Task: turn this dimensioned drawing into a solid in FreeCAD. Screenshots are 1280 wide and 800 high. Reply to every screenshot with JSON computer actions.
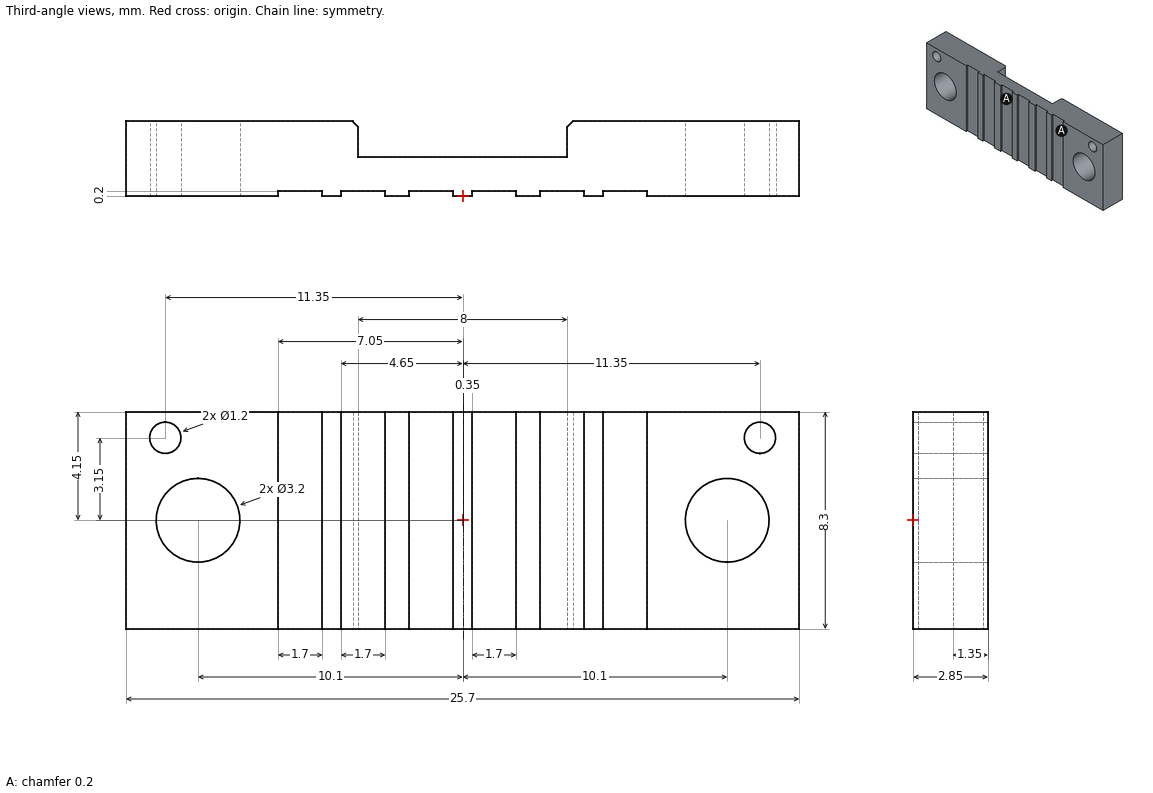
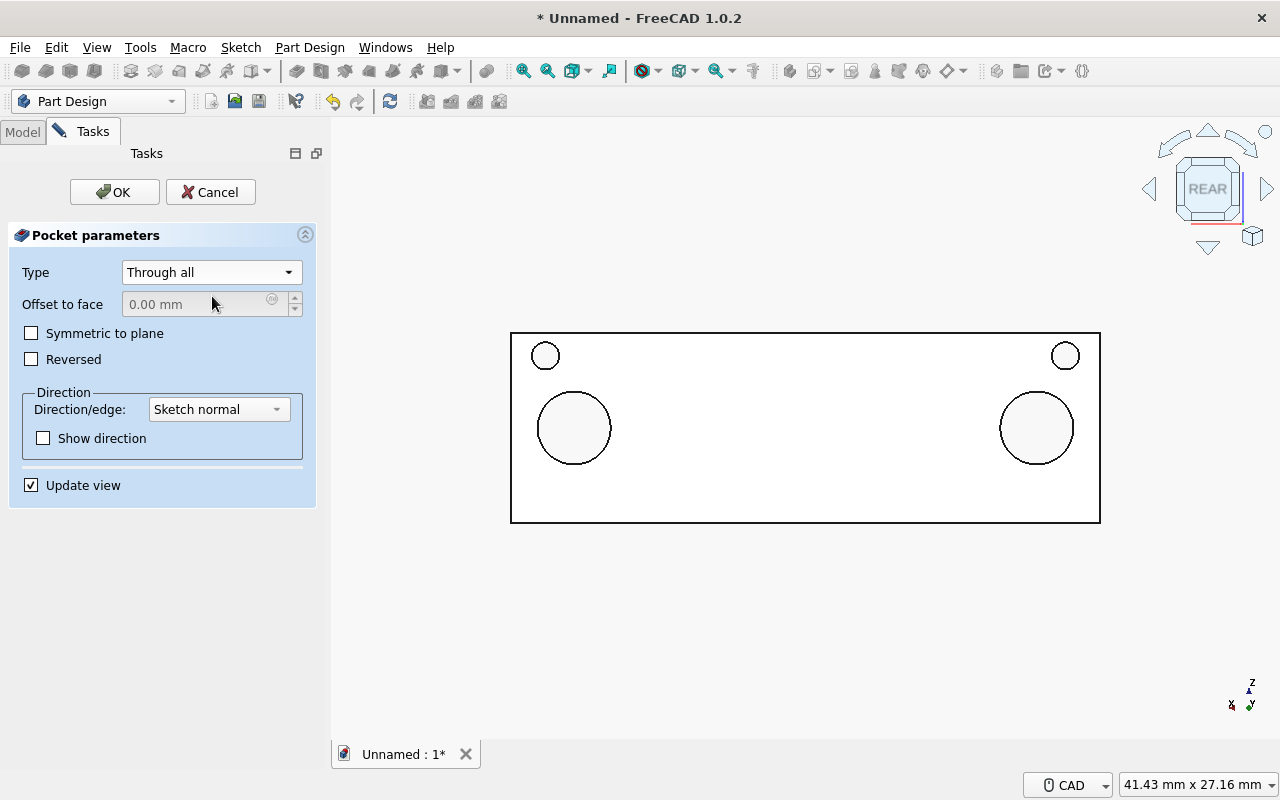
{"action": "left_click", "coordinate": [115, 192]}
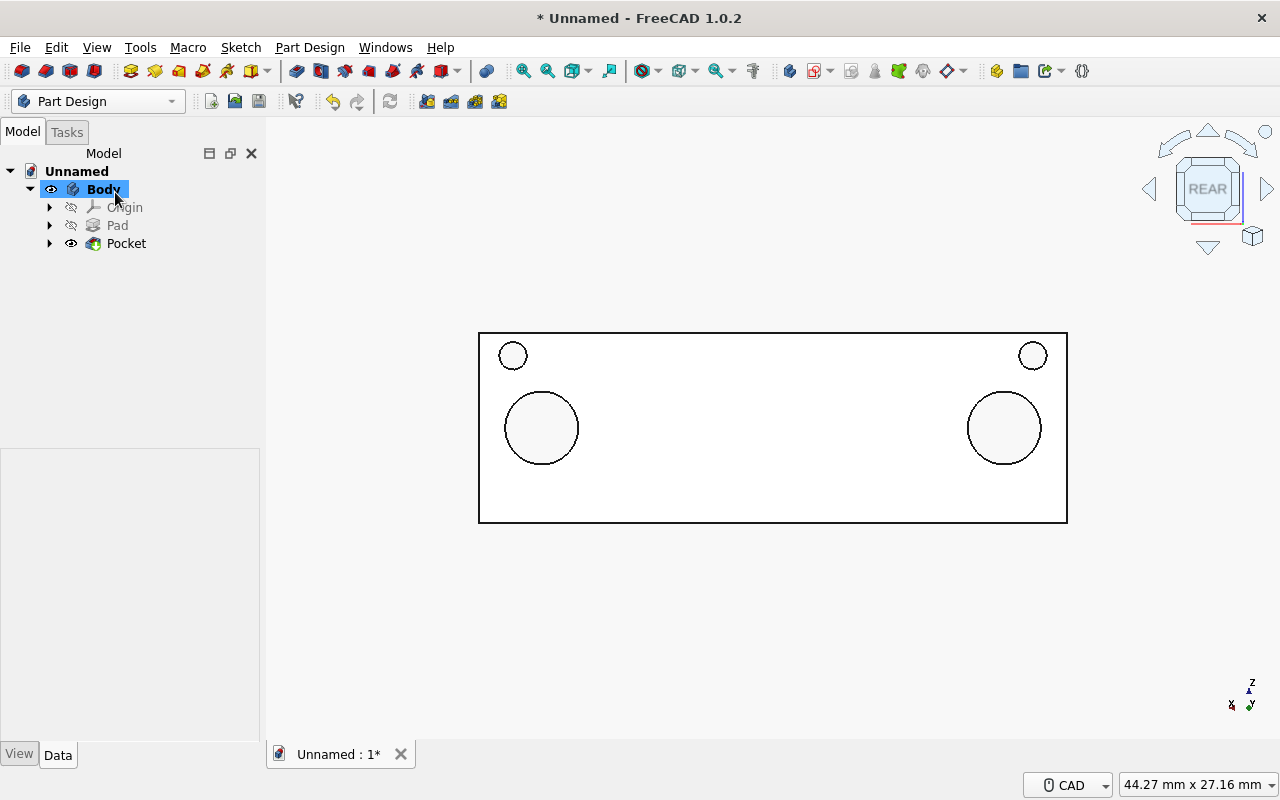
{"action": "key", "text": "0"}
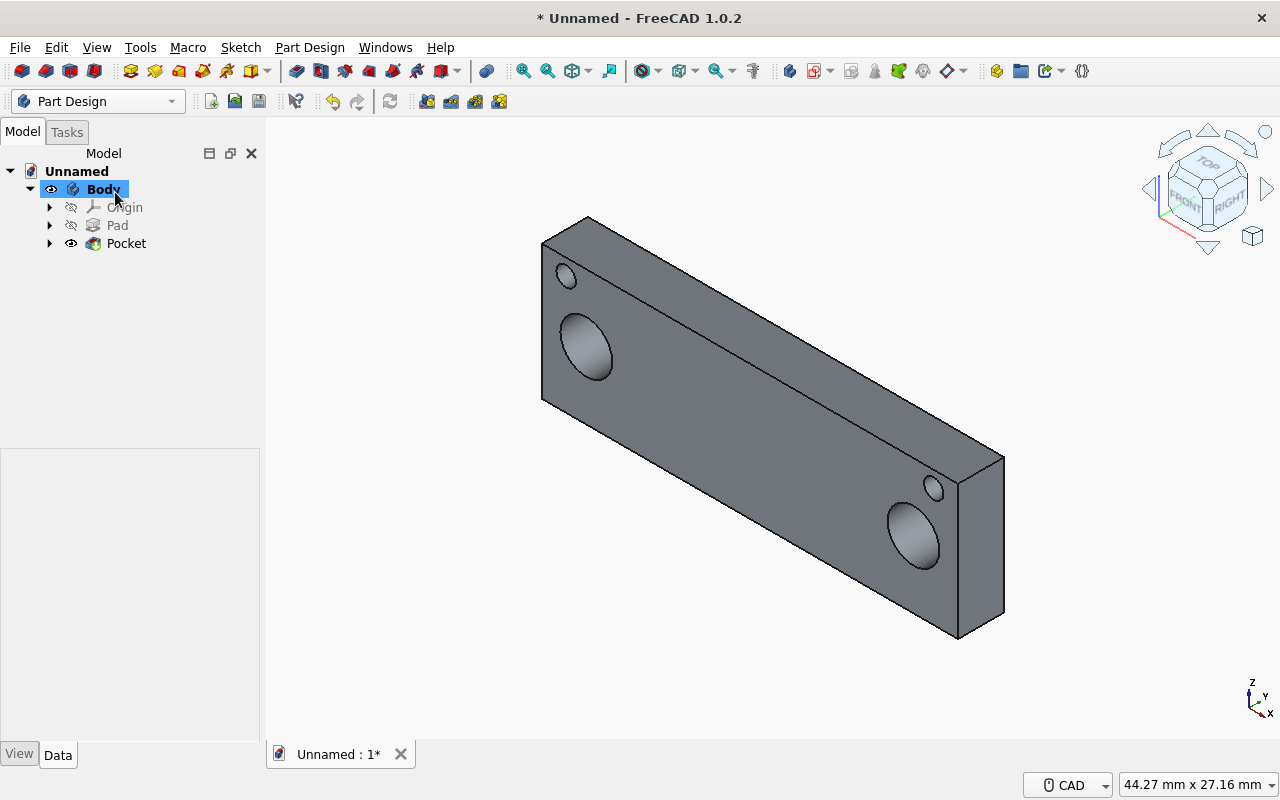
{"action": "left_click", "coordinate": [809, 475]}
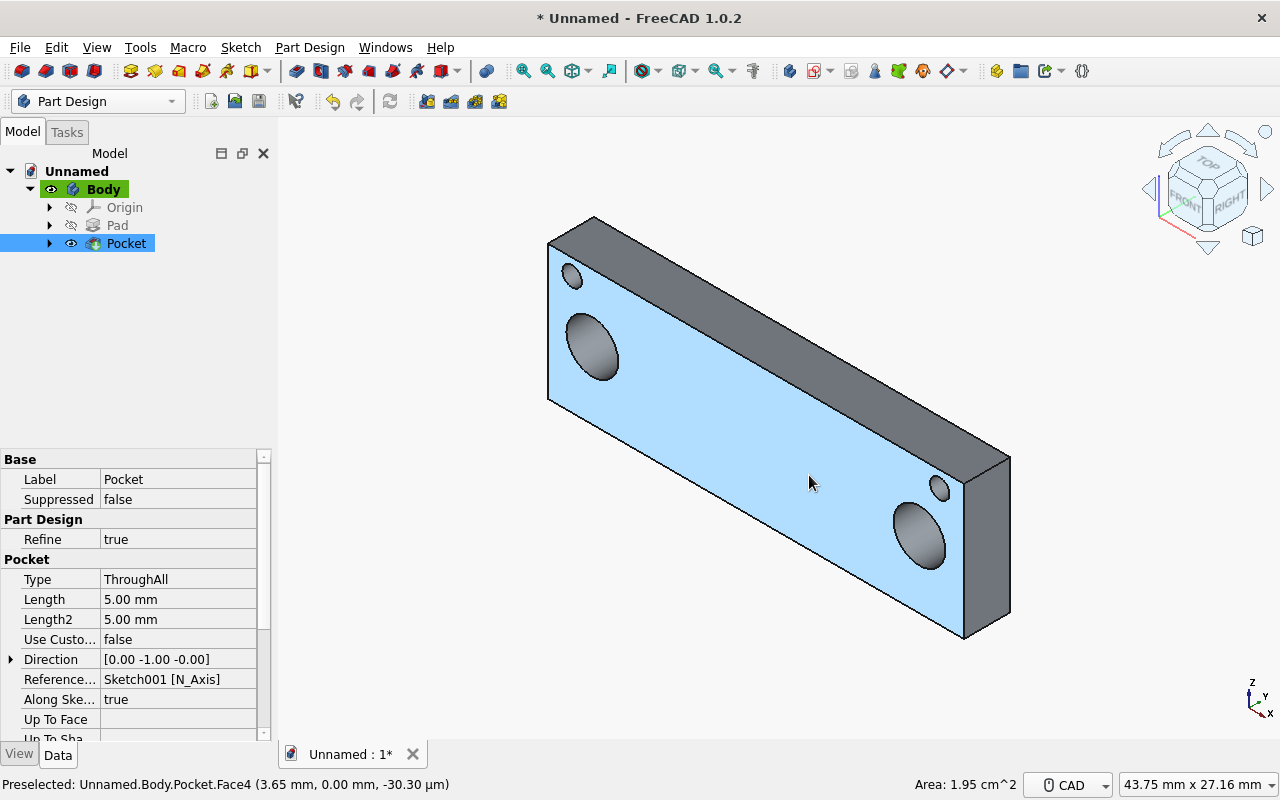
{"action": "left_click", "coordinate": [814, 72]}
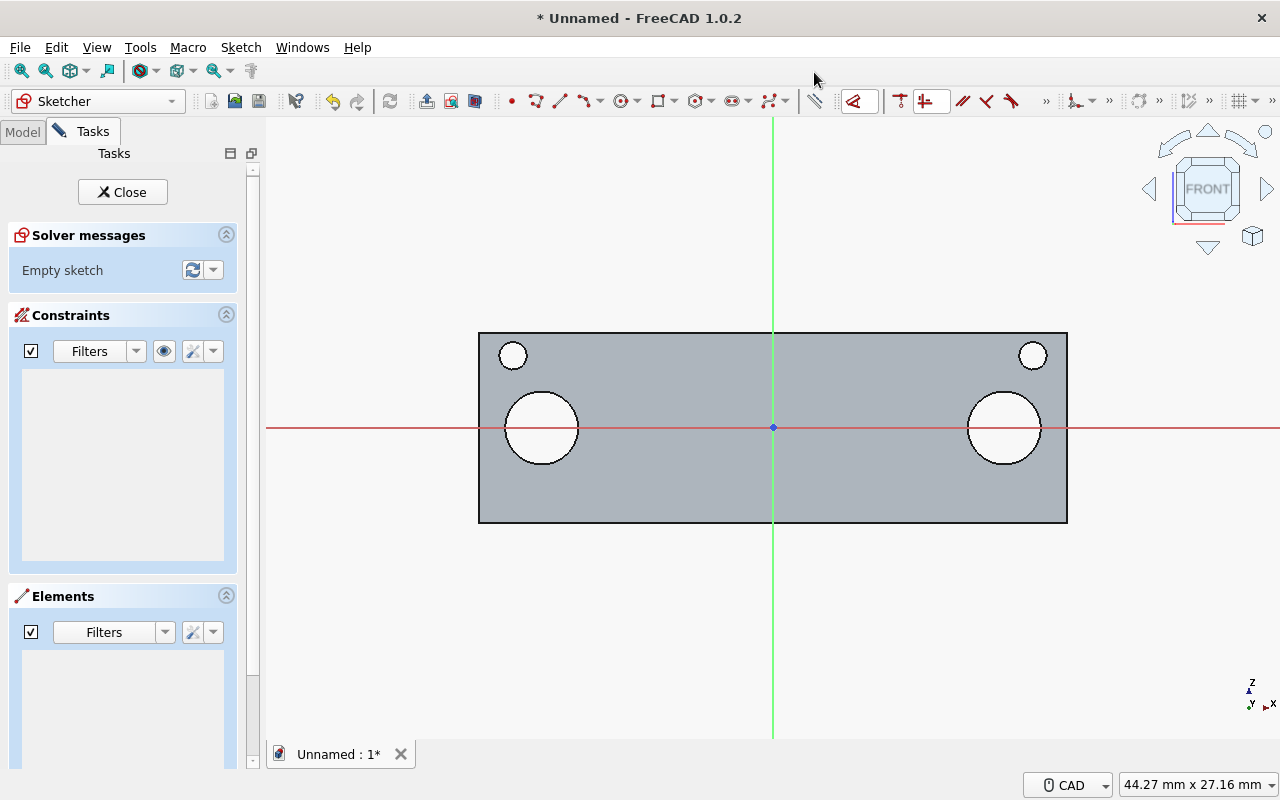
{"action": "scroll", "coordinate": [856, 428], "scroll_direction": "up", "scroll_amount": 3}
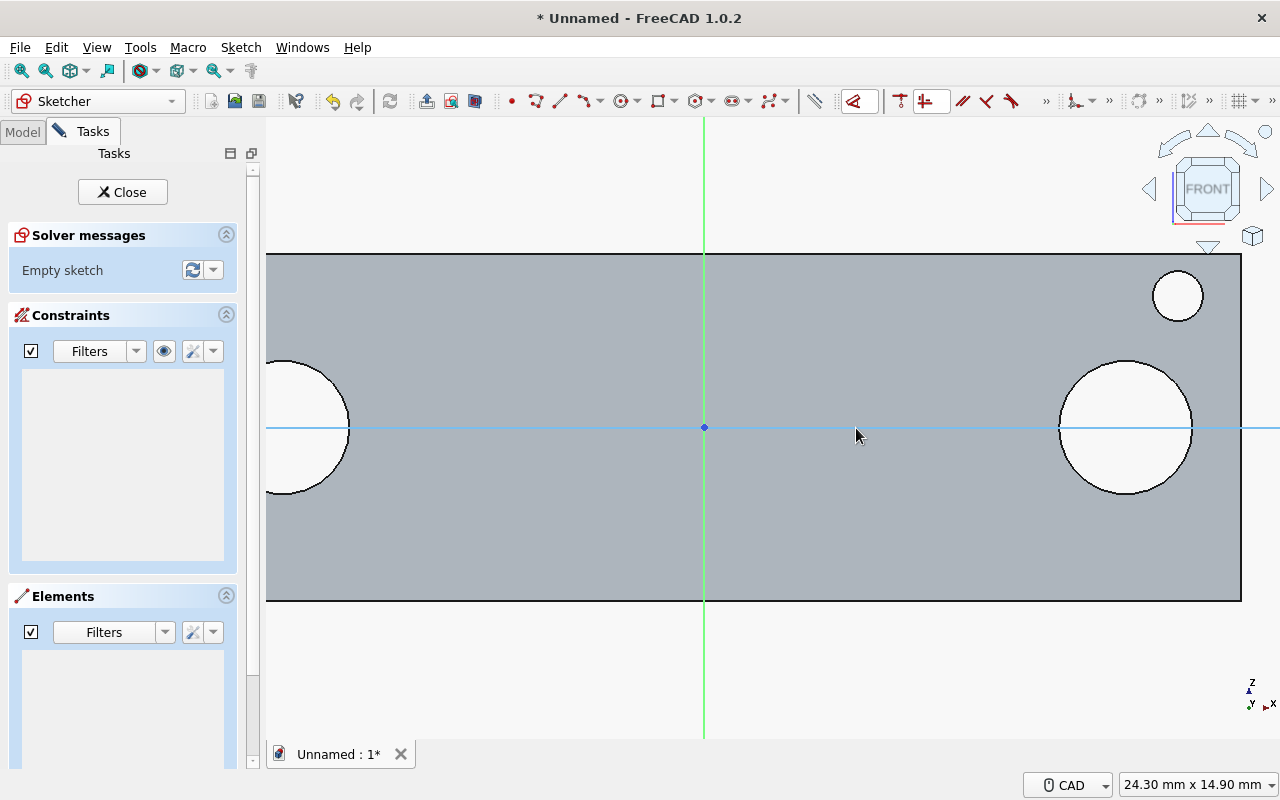
{"action": "key", "text": "g r"}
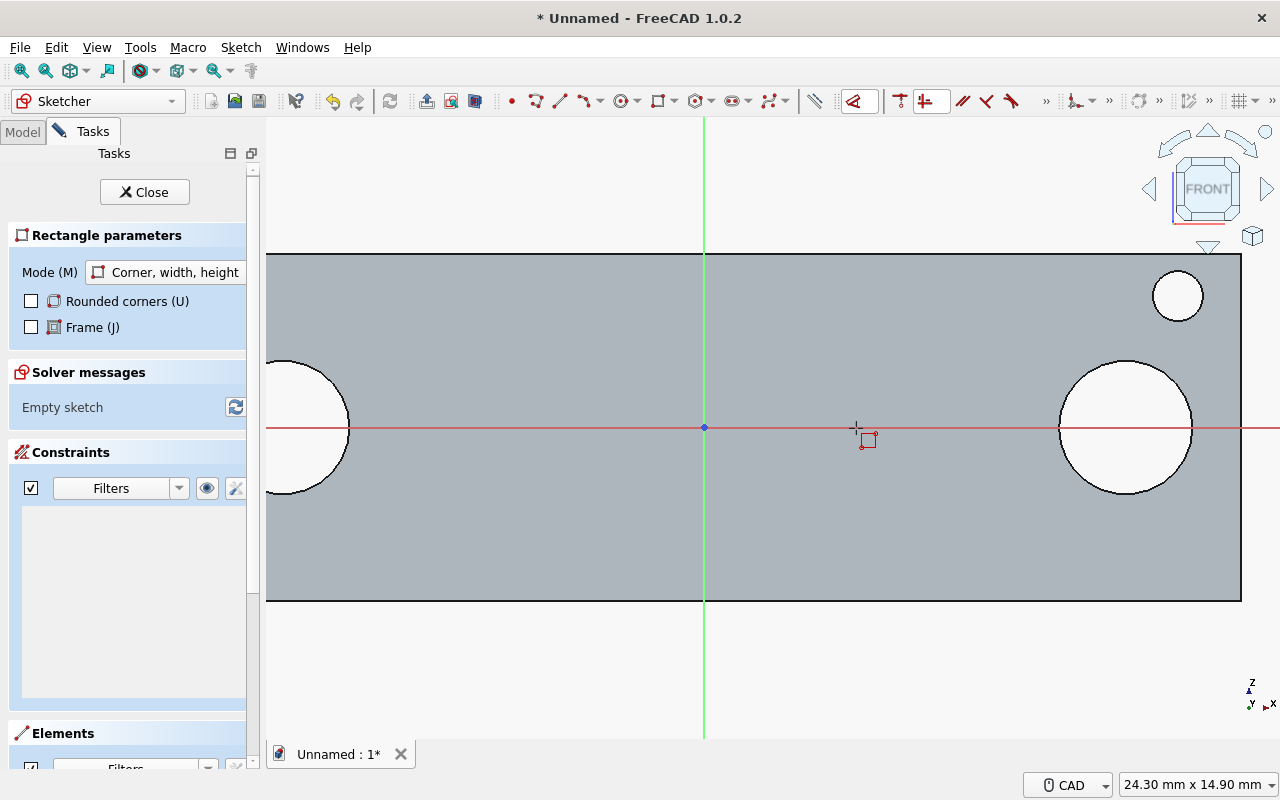
{"action": "left_click", "coordinate": [410, 254]}
{"action": "left_click", "coordinate": [481, 601]}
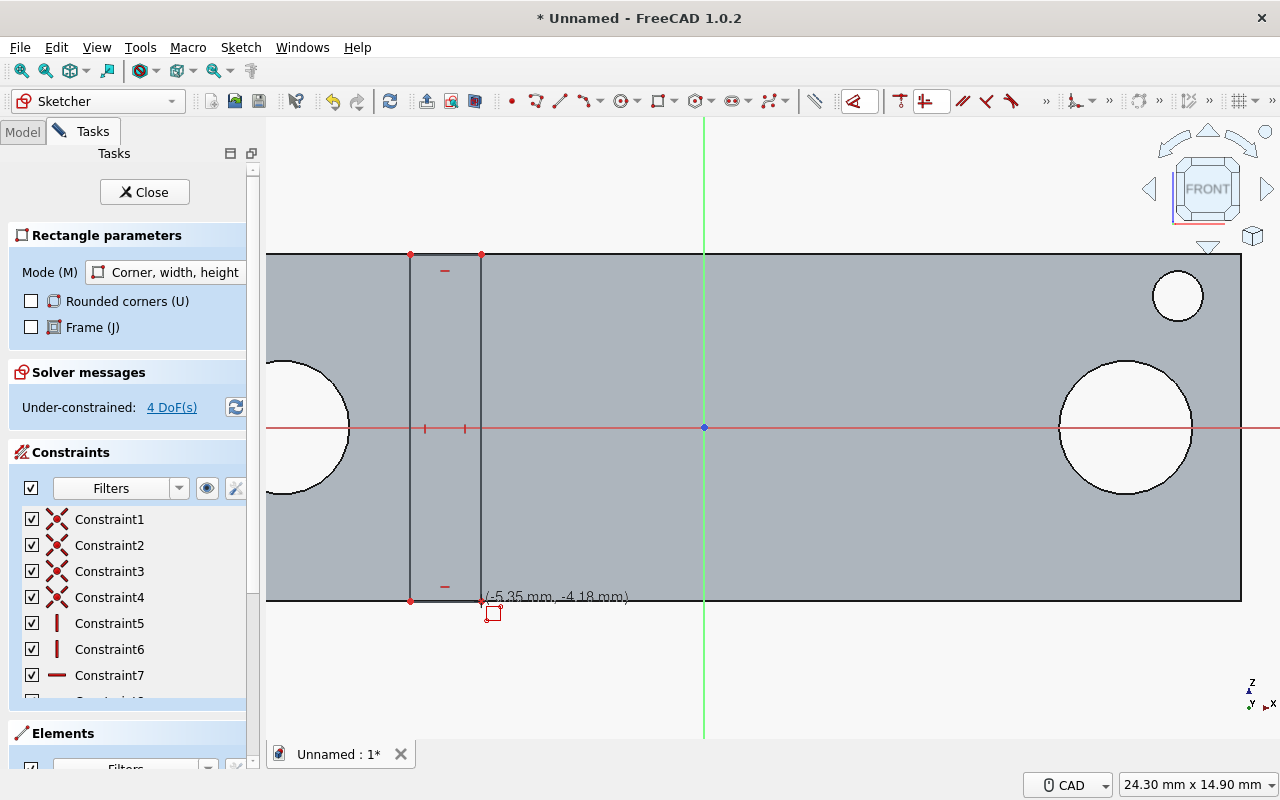
{"action": "left_click", "coordinate": [719, 254]}
{"action": "left_click", "coordinate": [790, 601]}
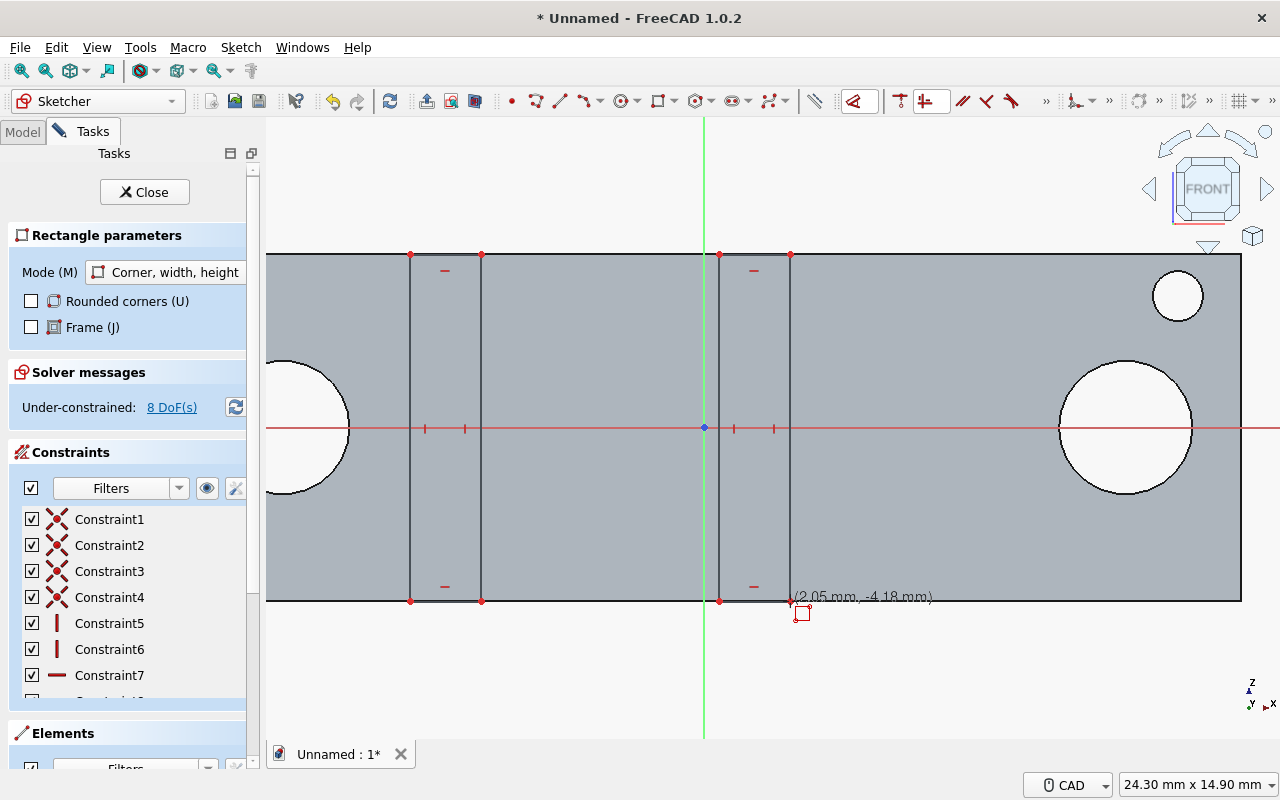
{"action": "left_click", "coordinate": [510, 254]}
{"action": "left_click", "coordinate": [581, 601]}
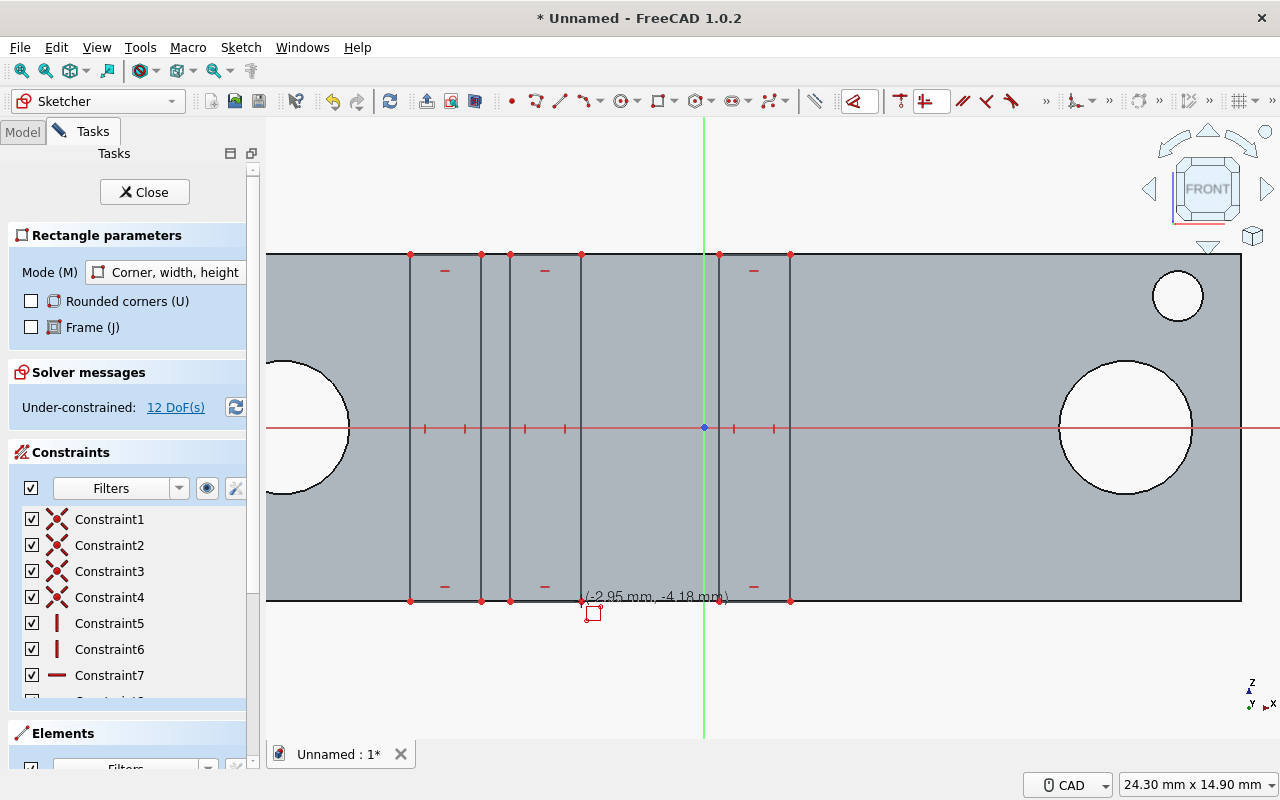
{"action": "left_click", "coordinate": [619, 254]}
{"action": "left_click", "coordinate": [690, 601]}